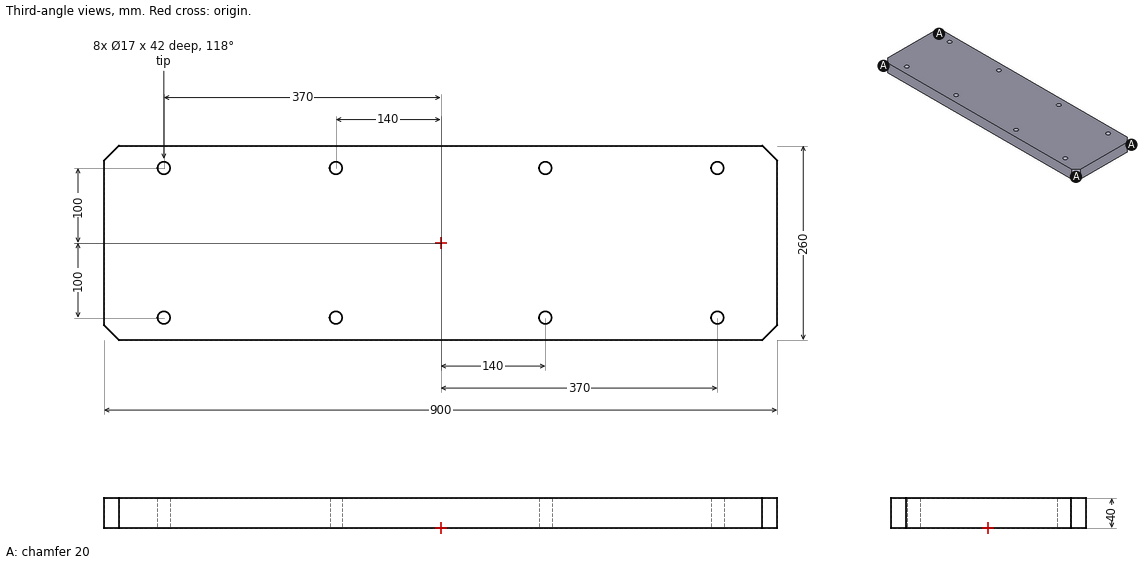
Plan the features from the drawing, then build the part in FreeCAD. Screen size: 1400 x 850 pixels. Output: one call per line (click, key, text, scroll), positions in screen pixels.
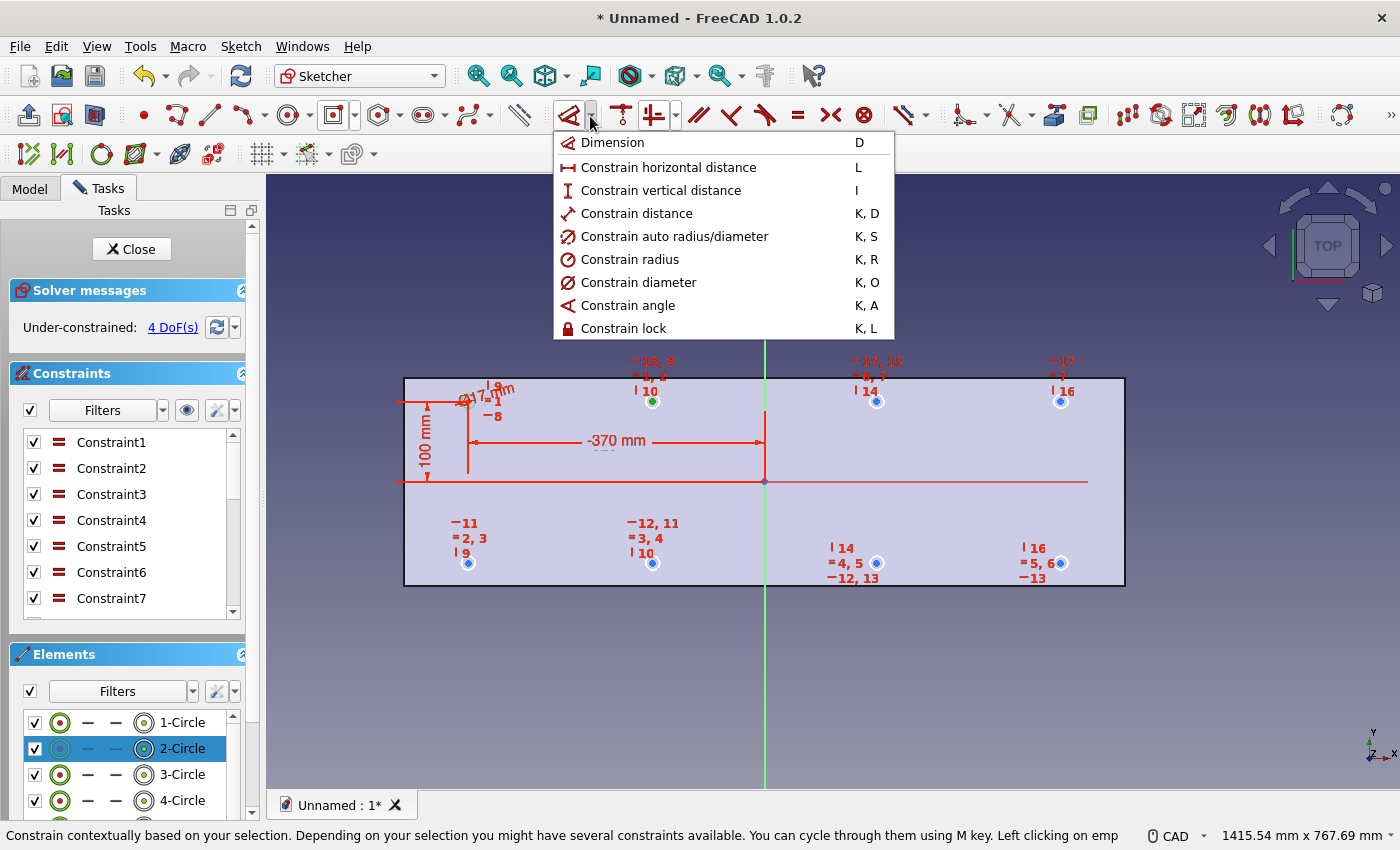
click(724, 168)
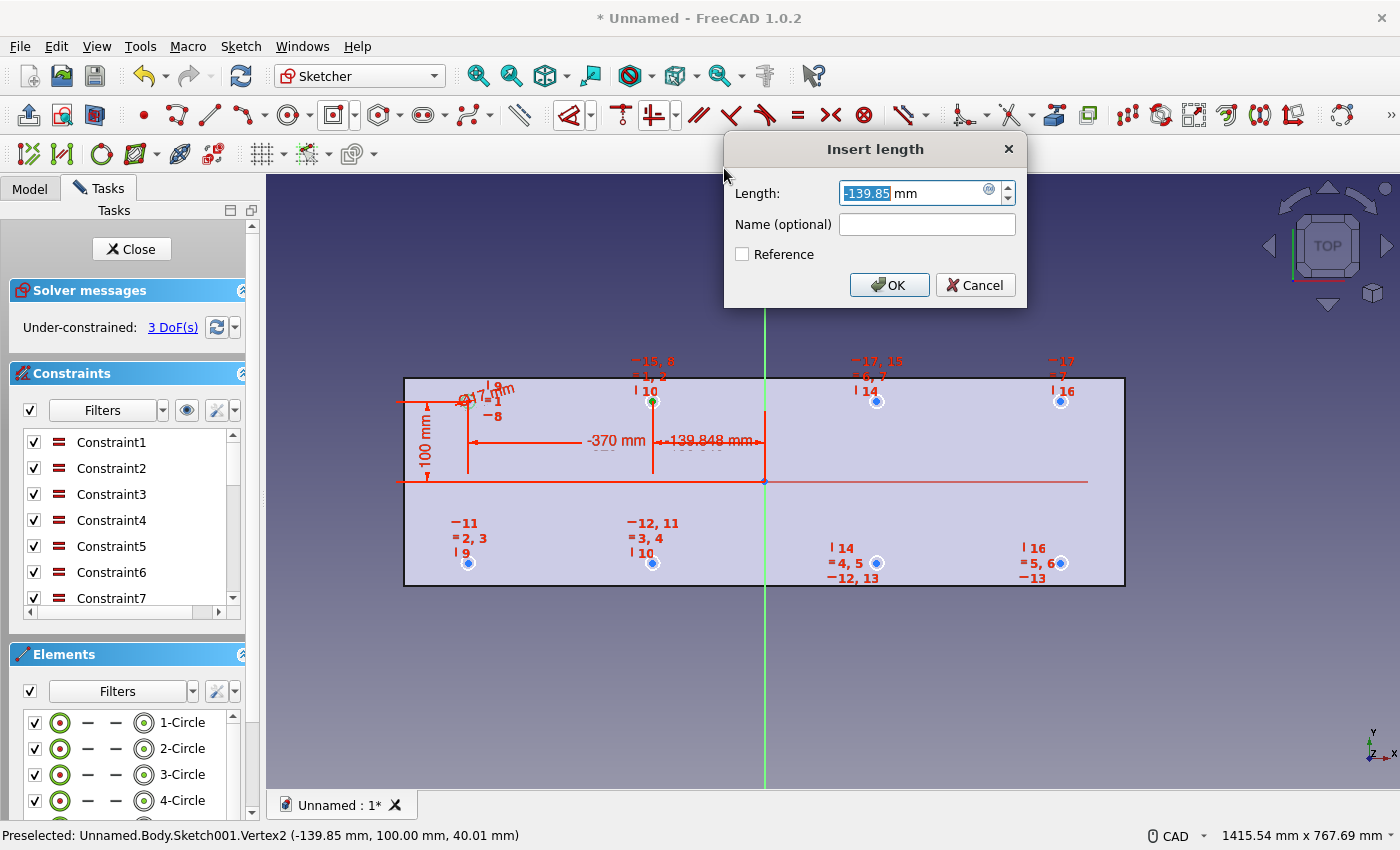
text(-140)
key(Return)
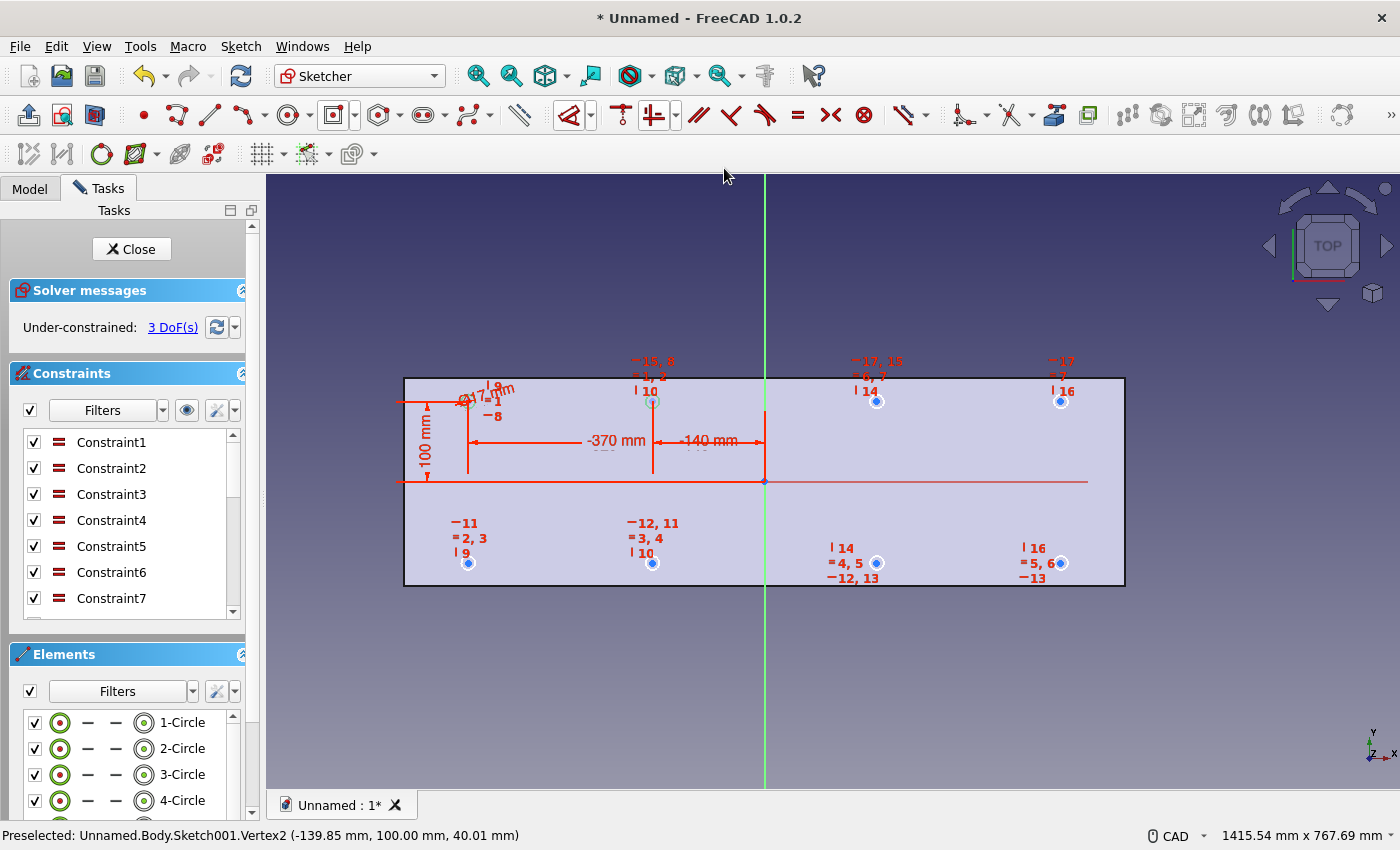
click(468, 563)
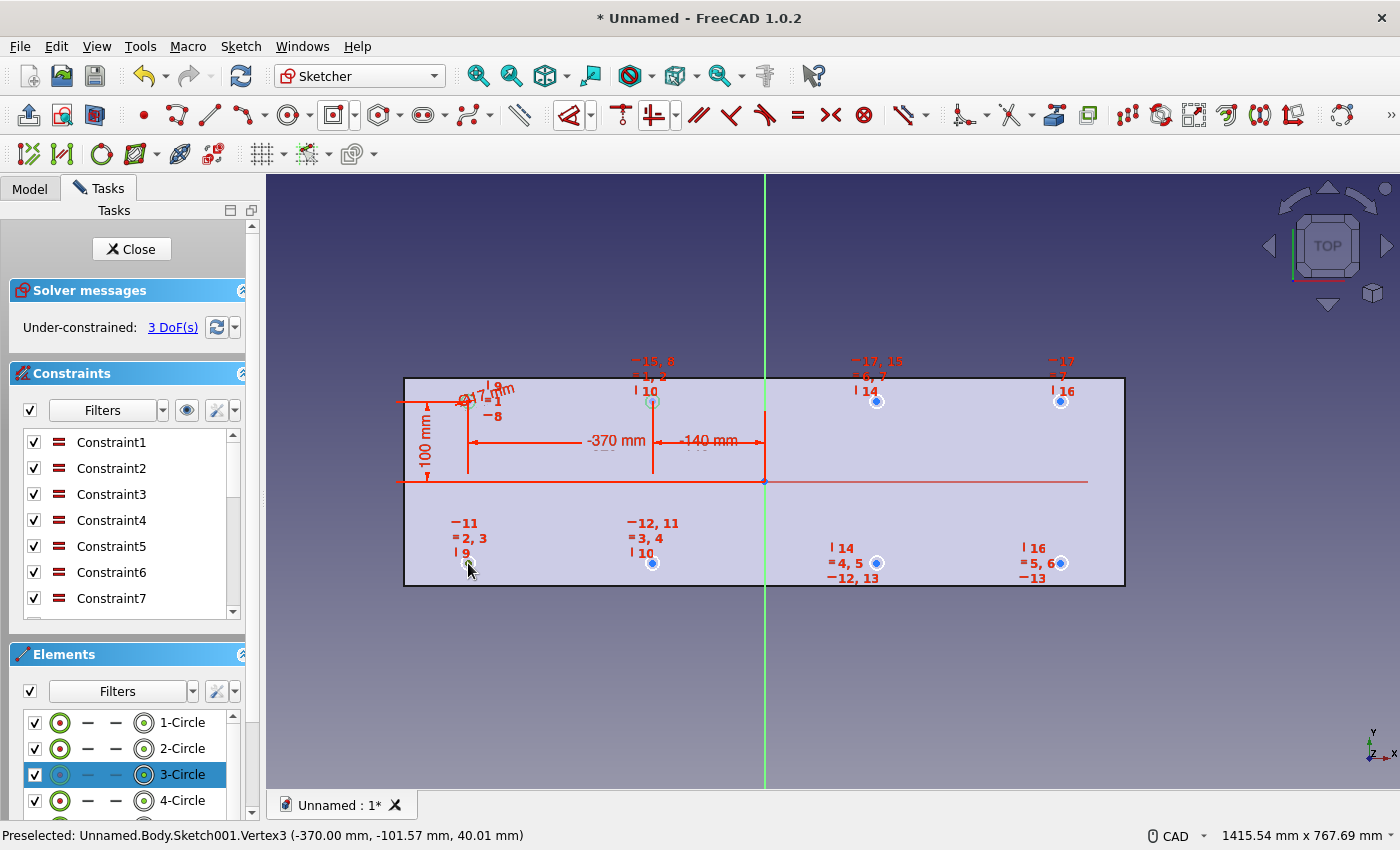
click(590, 116)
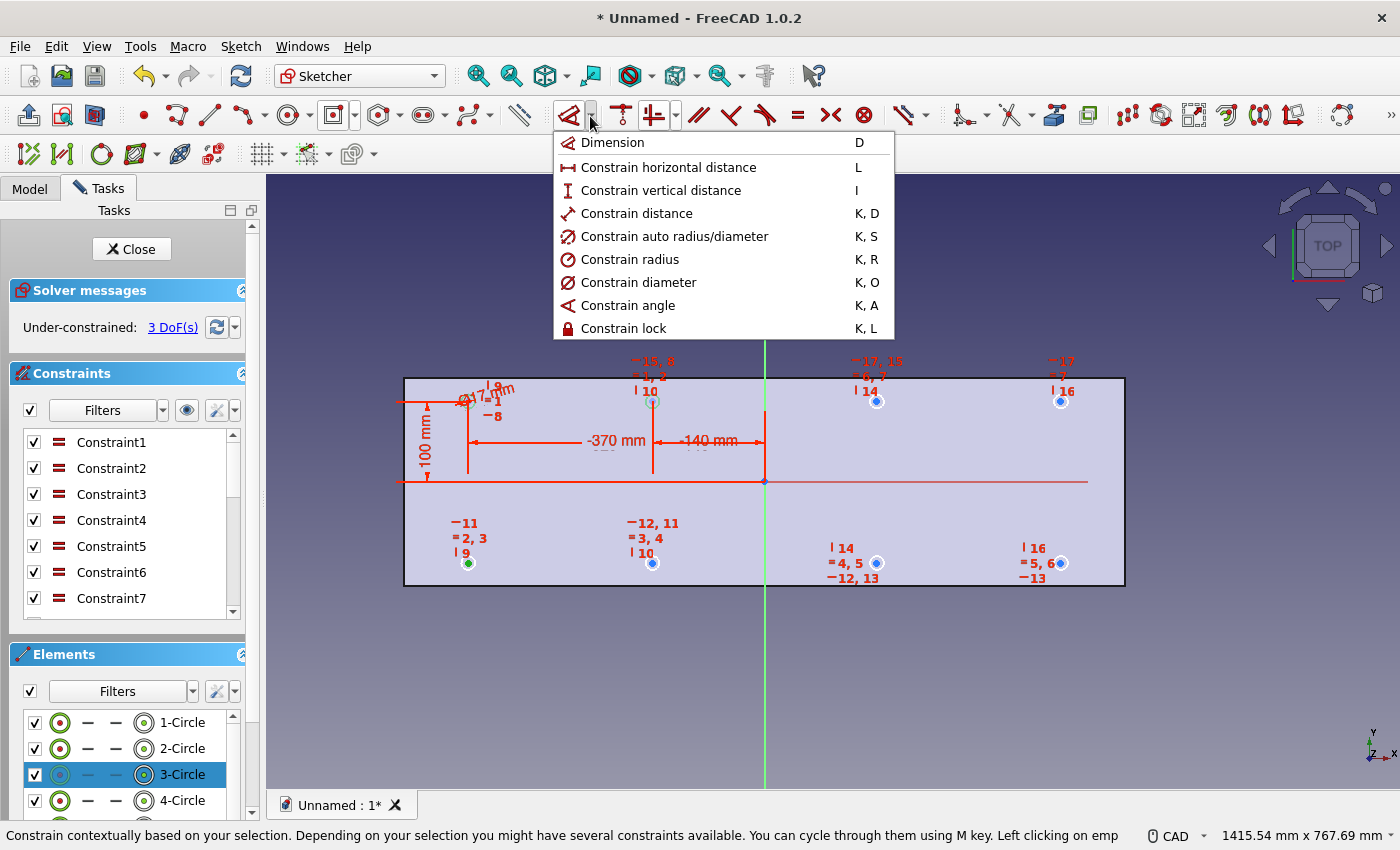
click(724, 190)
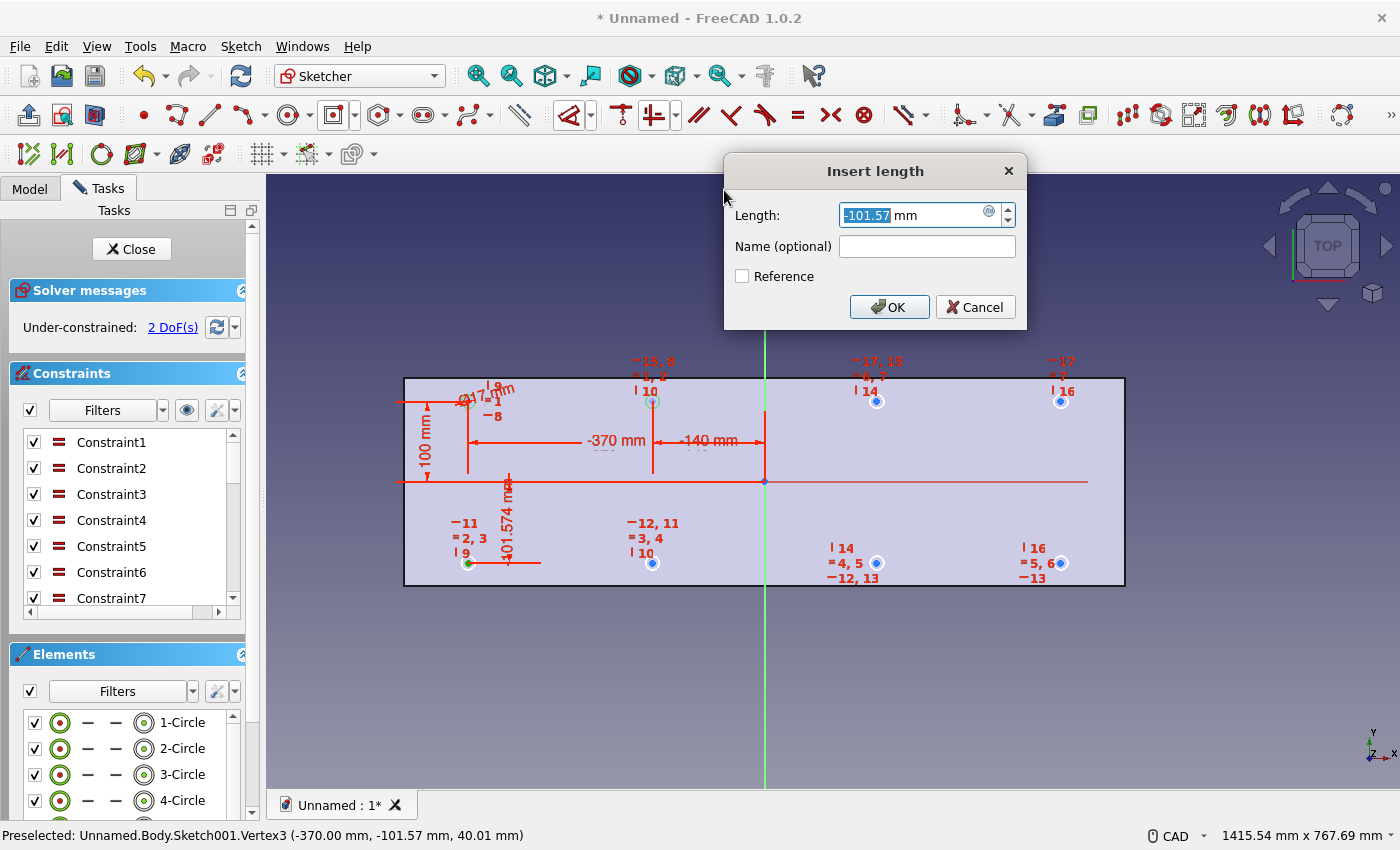
text(-100)
key(Return)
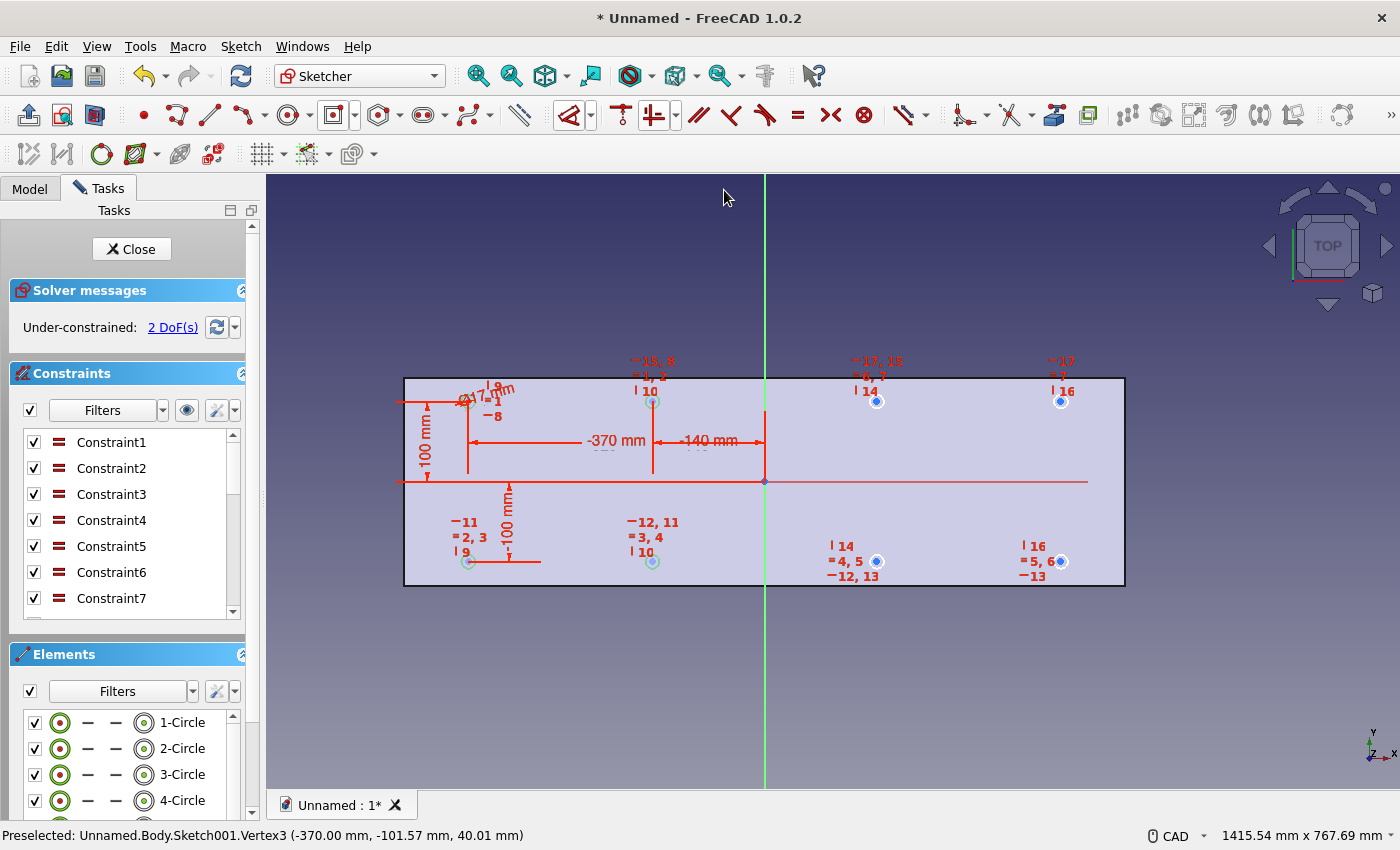
click(877, 562)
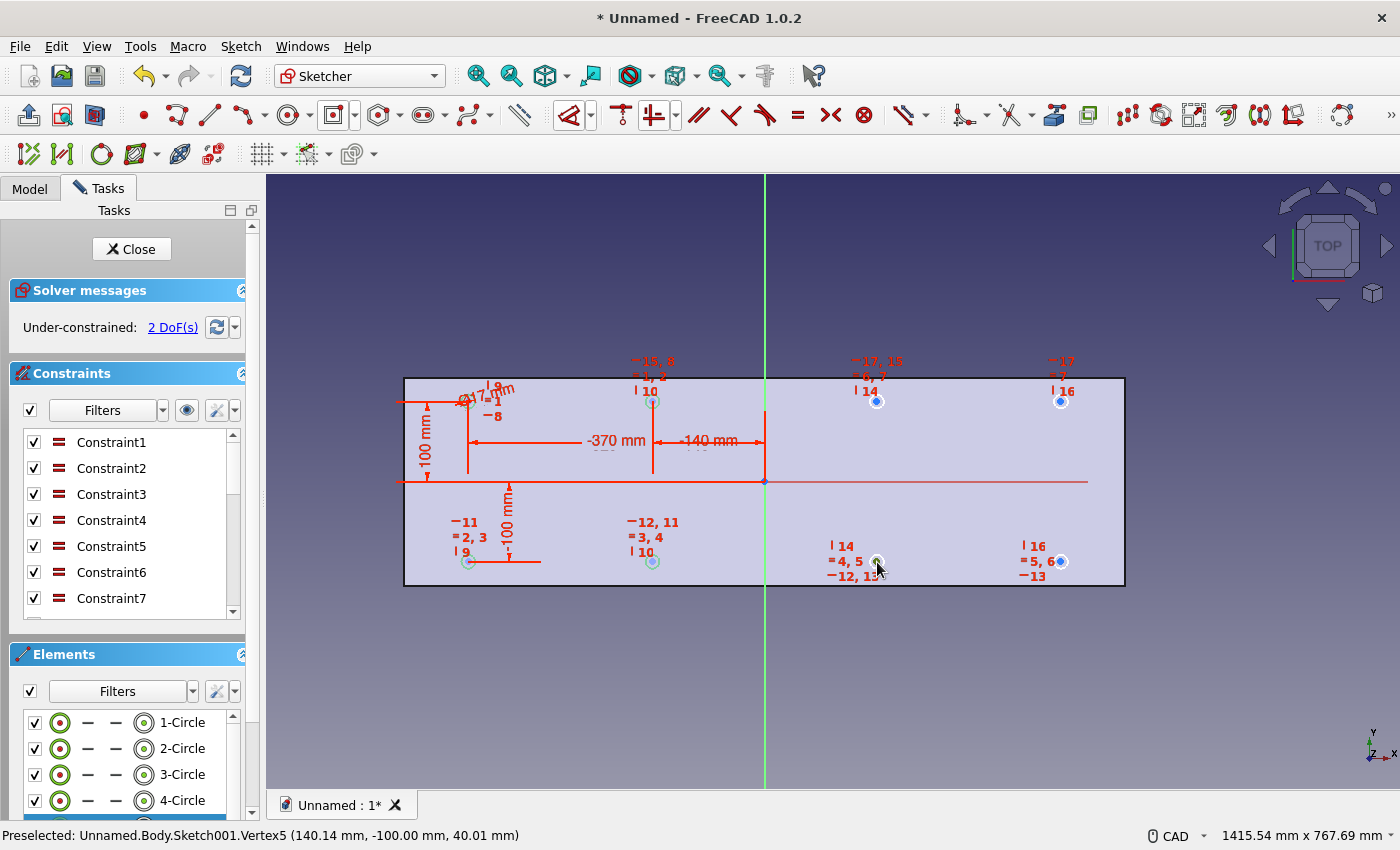
key(l)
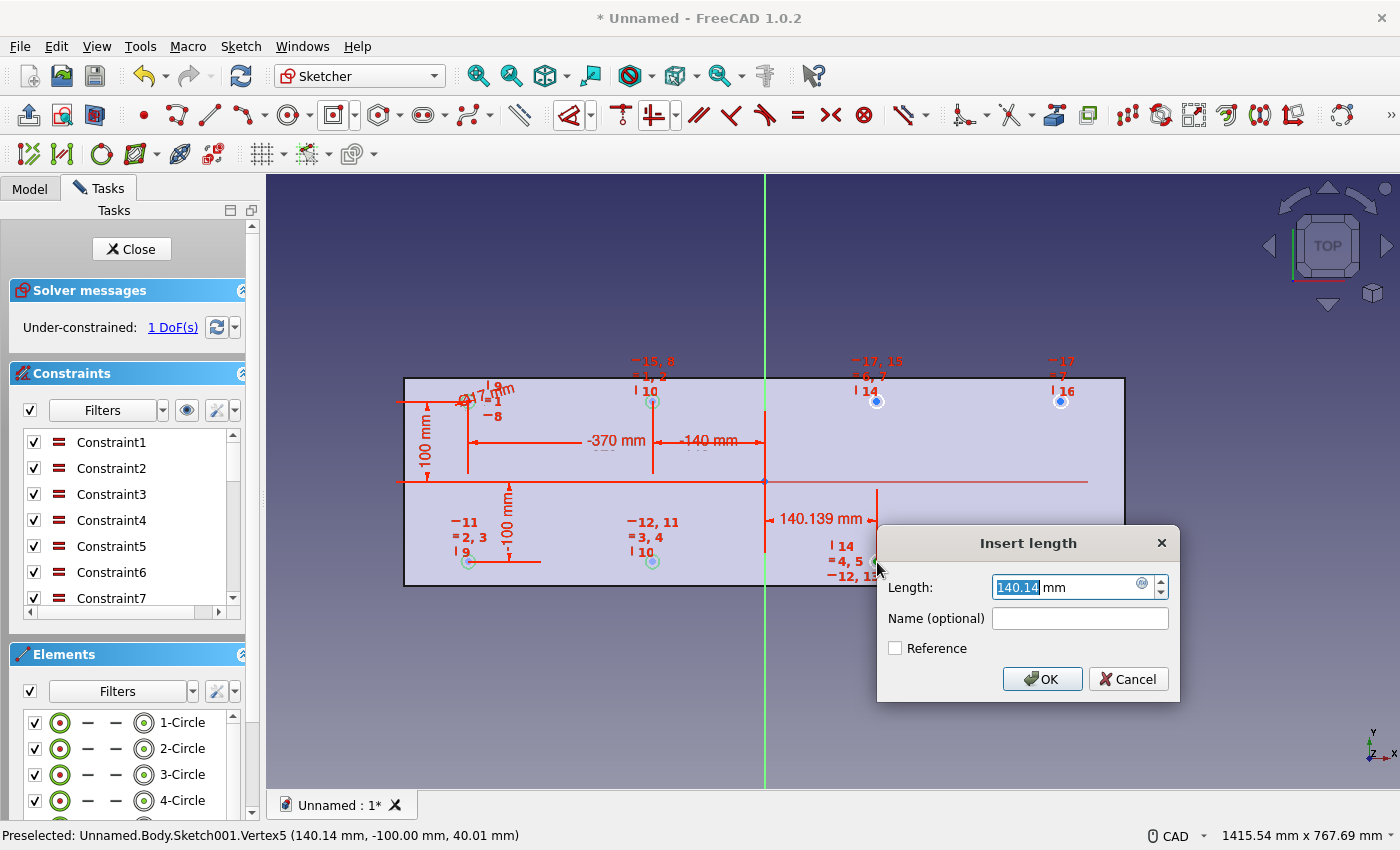
text(140)
key(Return)